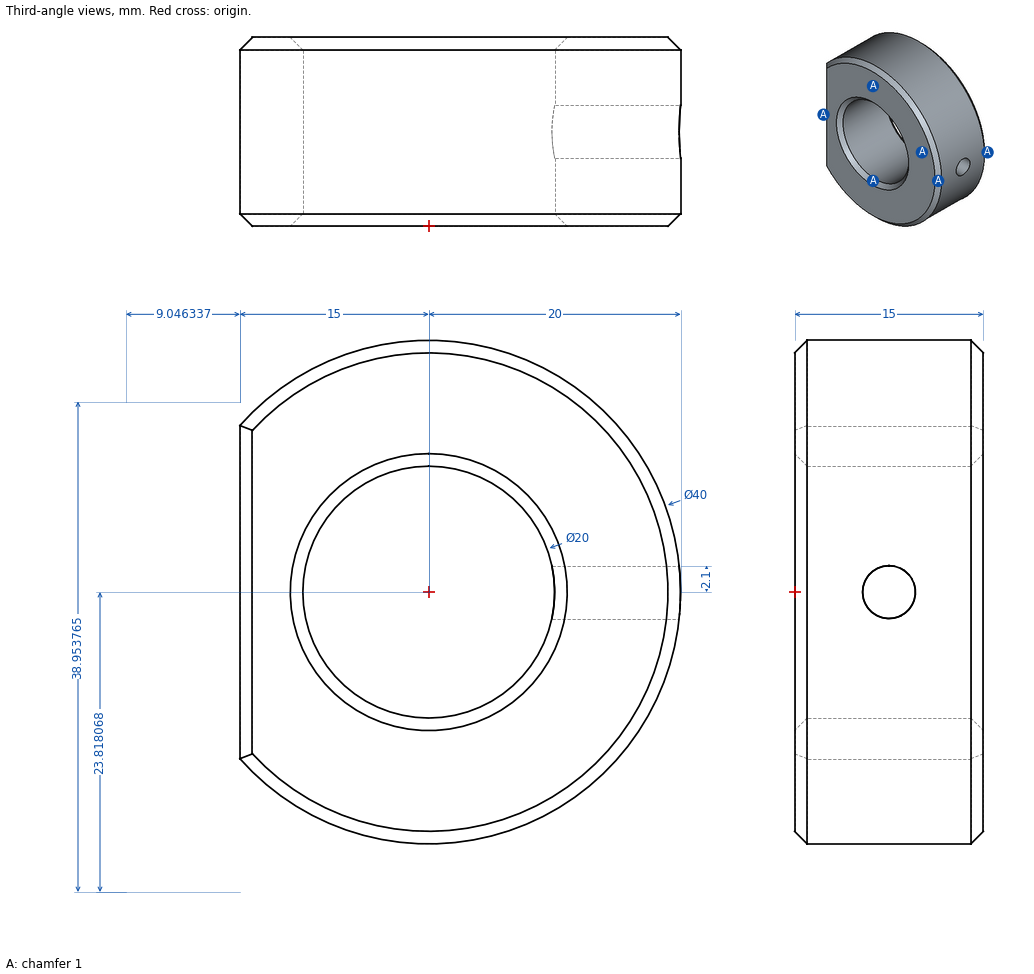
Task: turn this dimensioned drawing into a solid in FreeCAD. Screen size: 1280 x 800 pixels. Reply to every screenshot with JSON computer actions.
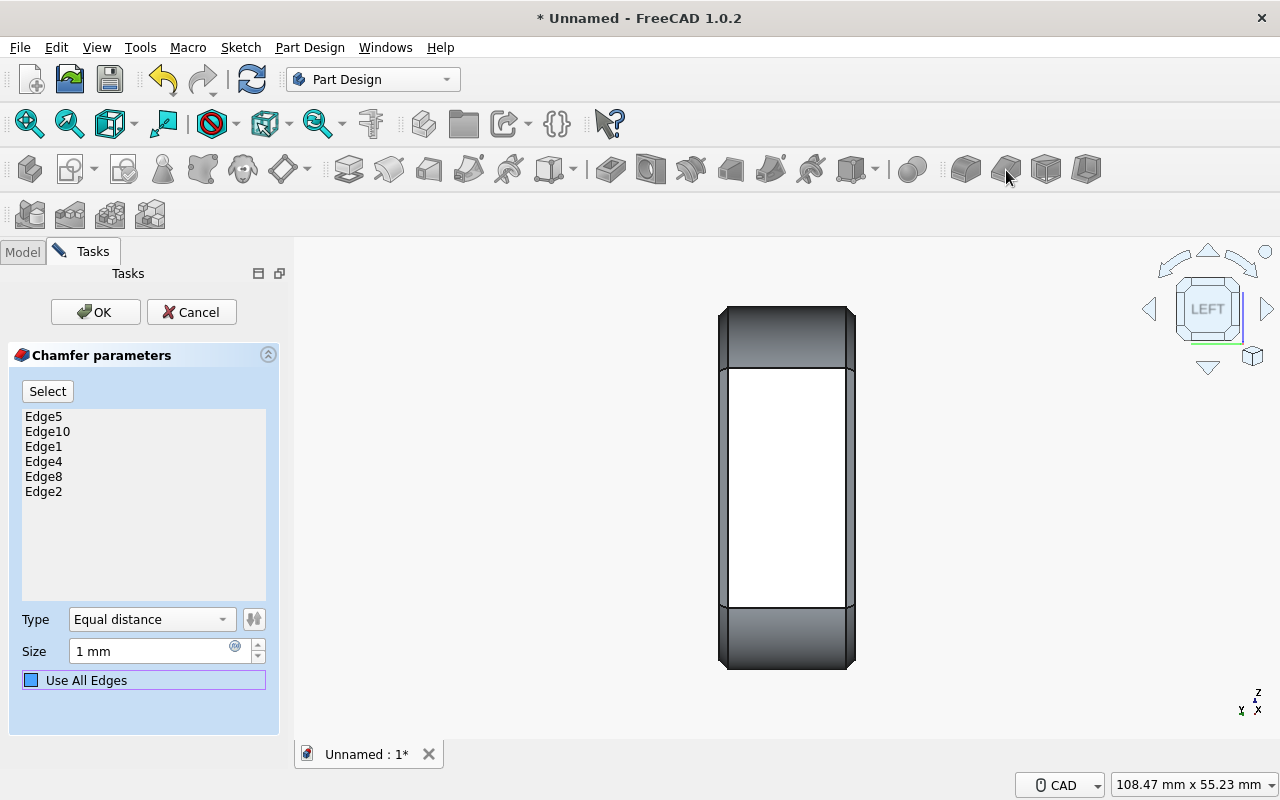
{"action": "left_click", "coordinate": [96, 312]}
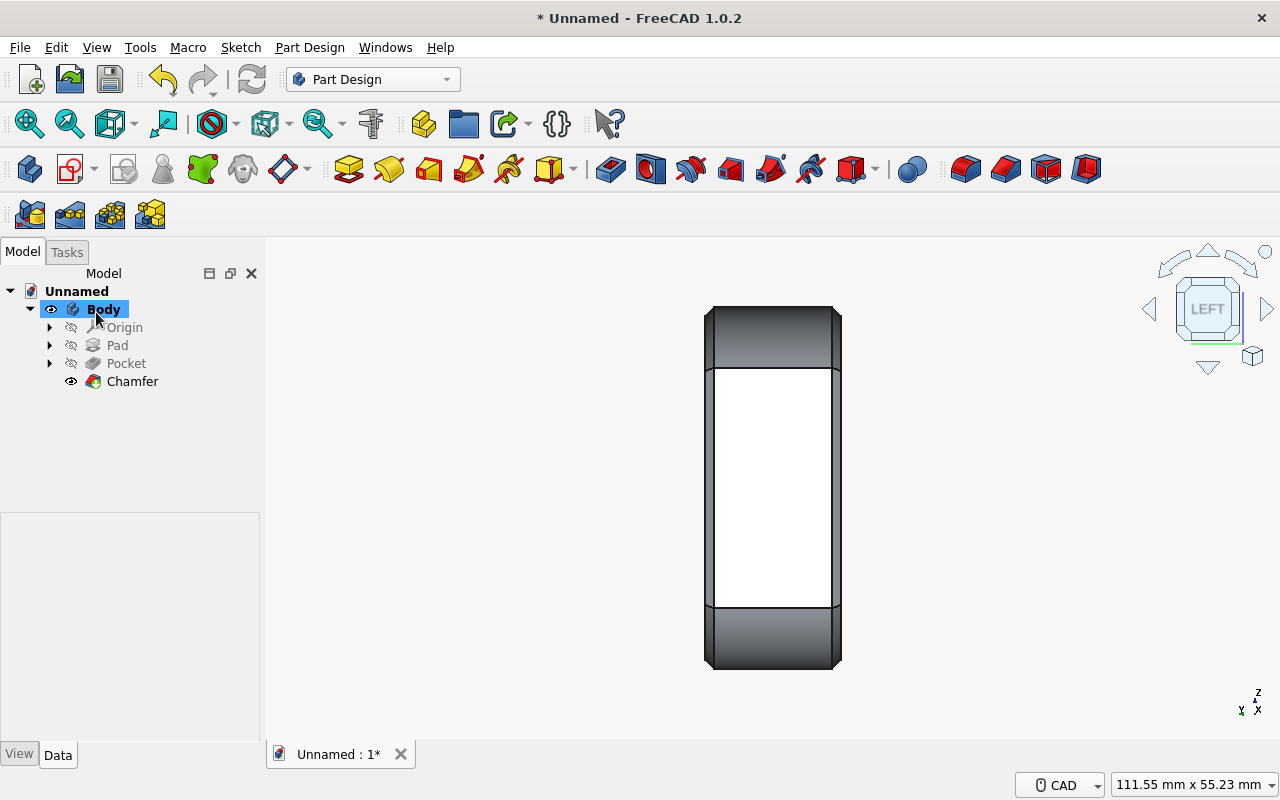
{"action": "left_click", "coordinate": [50, 327]}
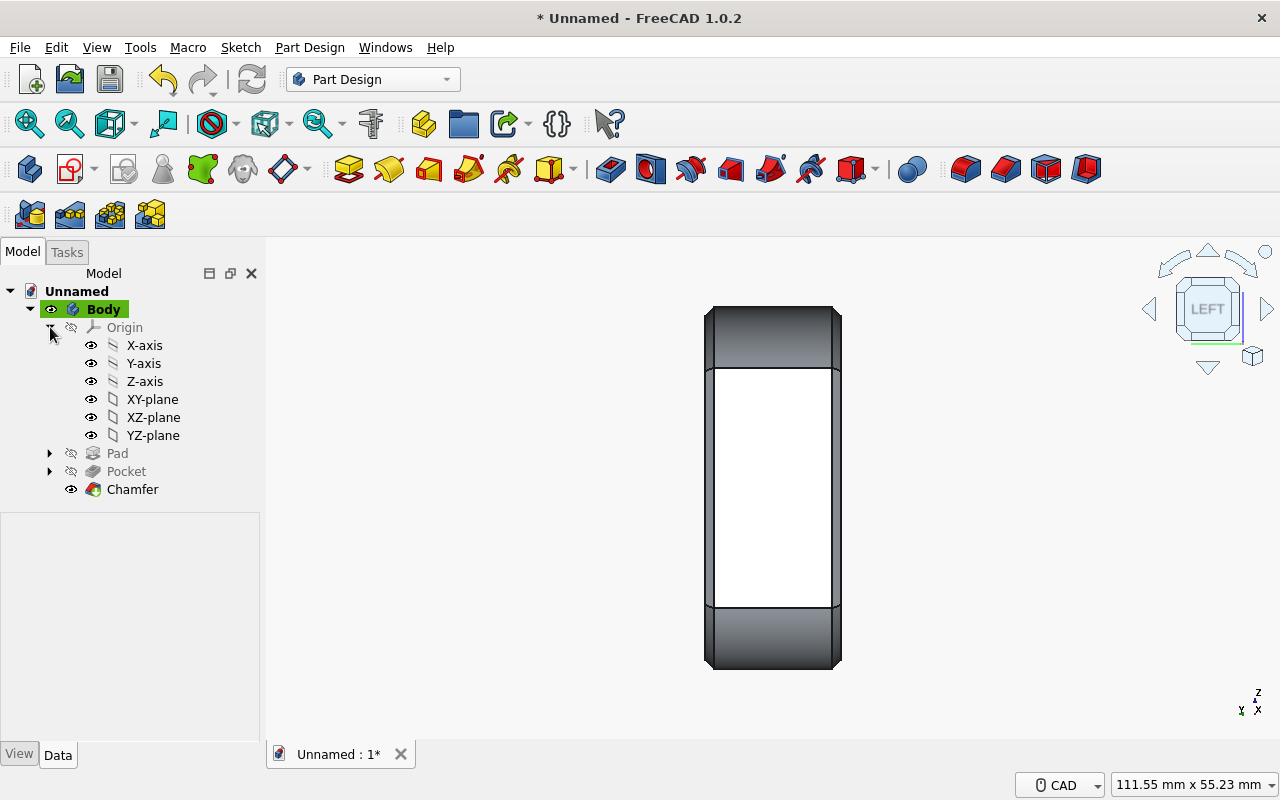
{"action": "left_click", "coordinate": [136, 417]}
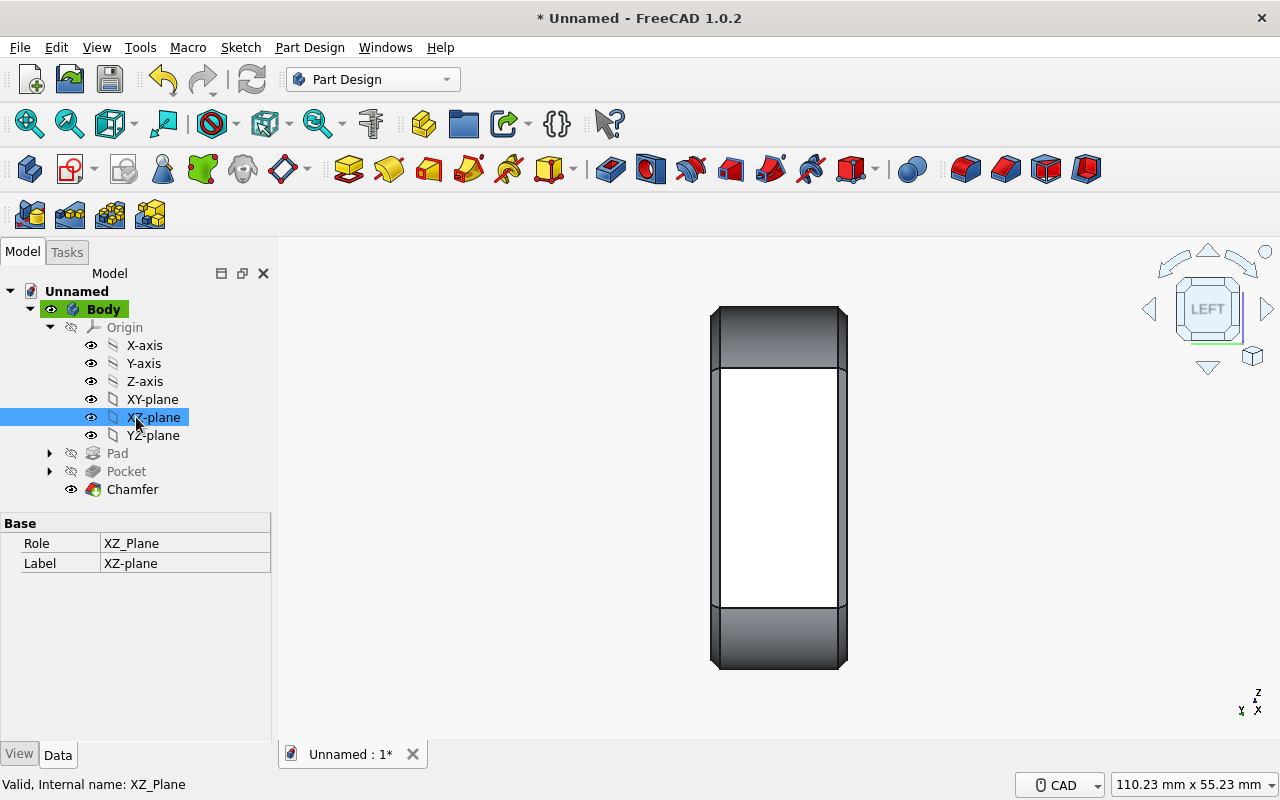
{"action": "left_click", "coordinate": [284, 170]}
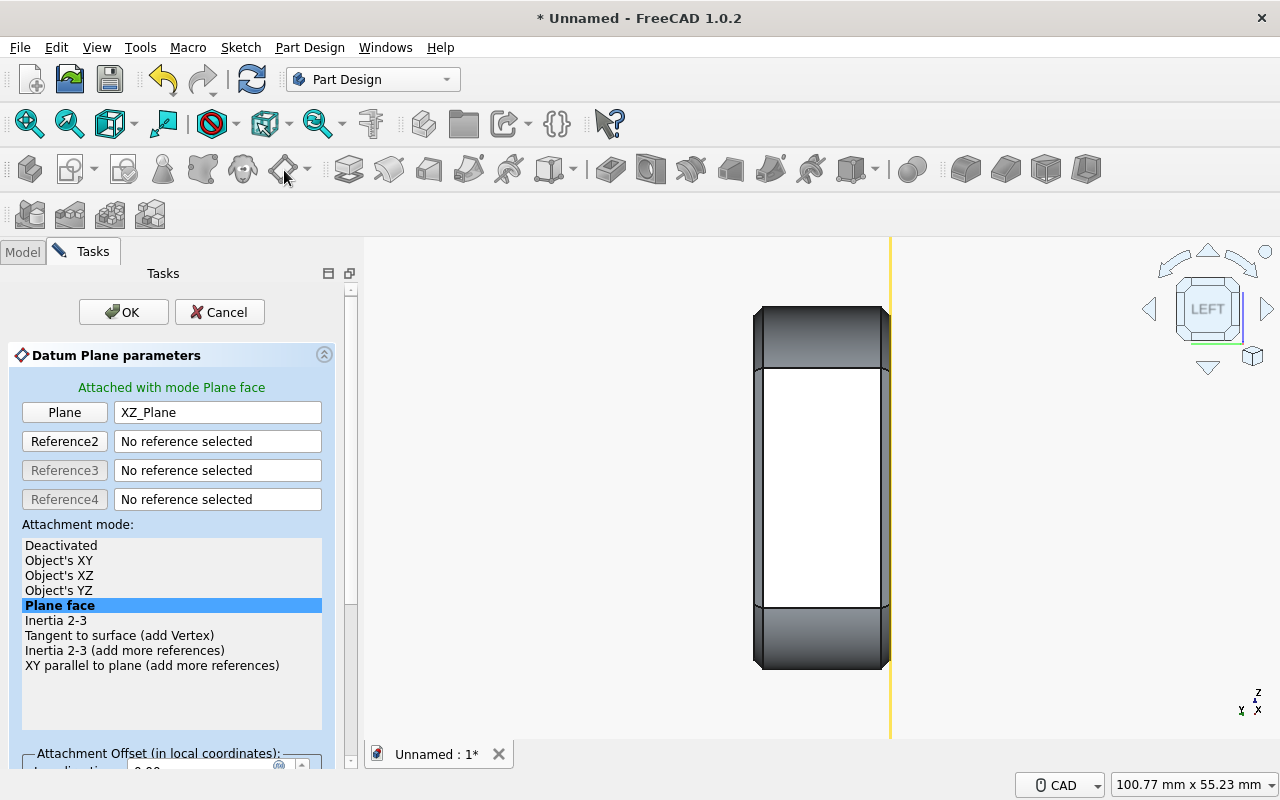
{"action": "scroll", "coordinate": [351, 526], "scroll_direction": "down", "scroll_amount": 3}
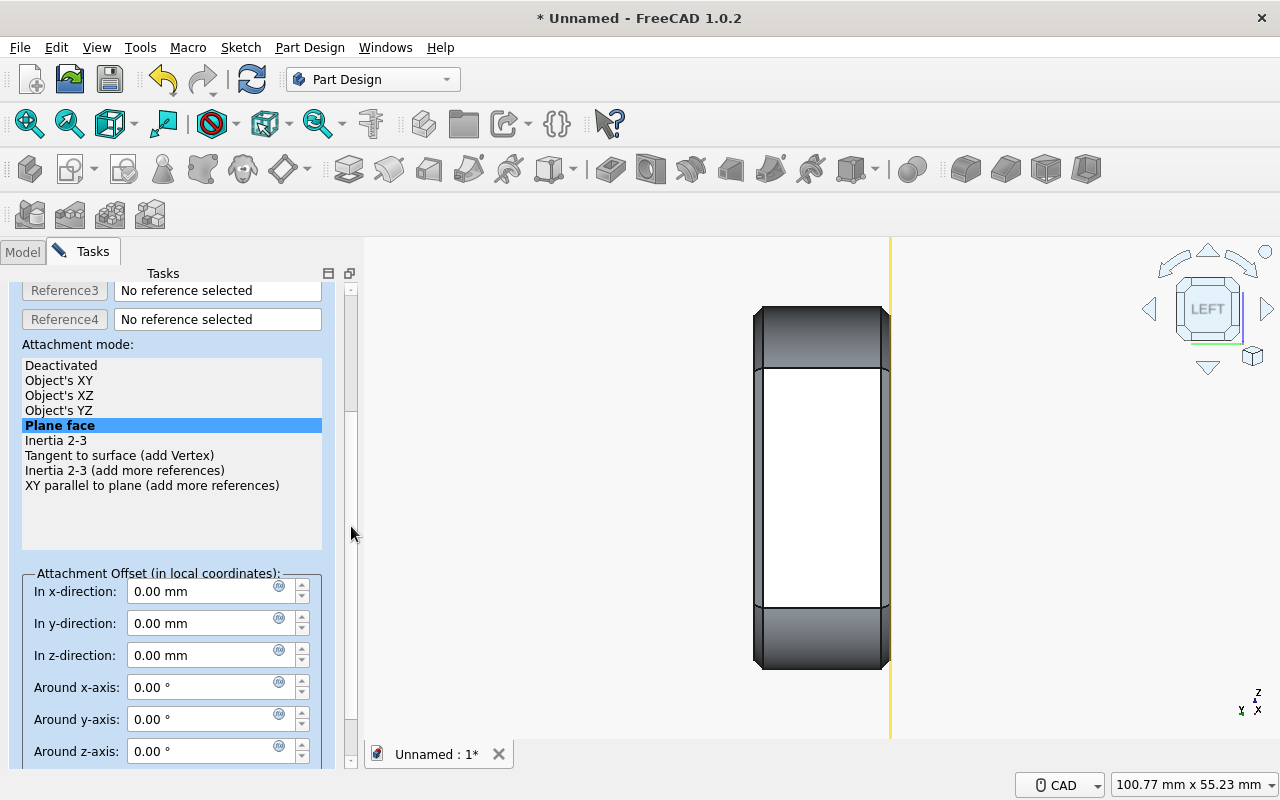
{"action": "triple_click", "coordinate": [210, 655]}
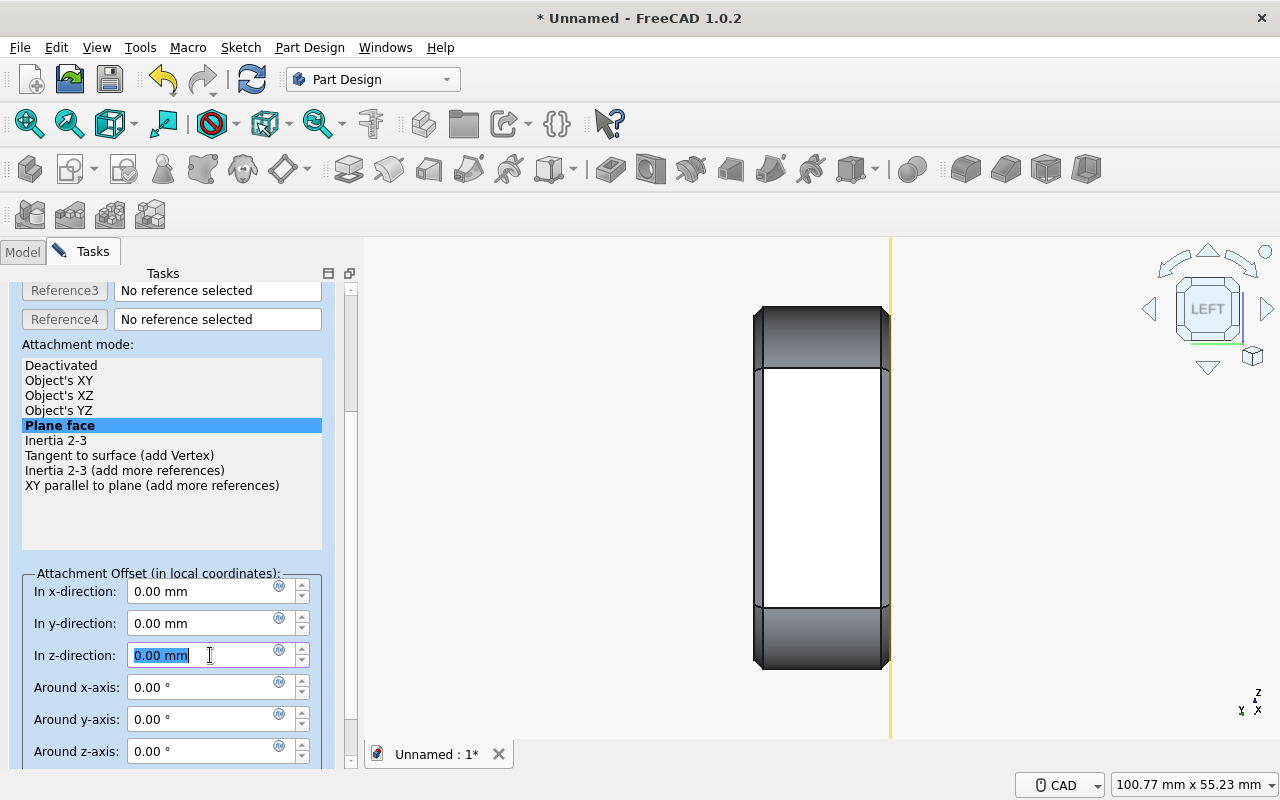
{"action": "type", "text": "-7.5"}
{"action": "key", "text": "Tab"}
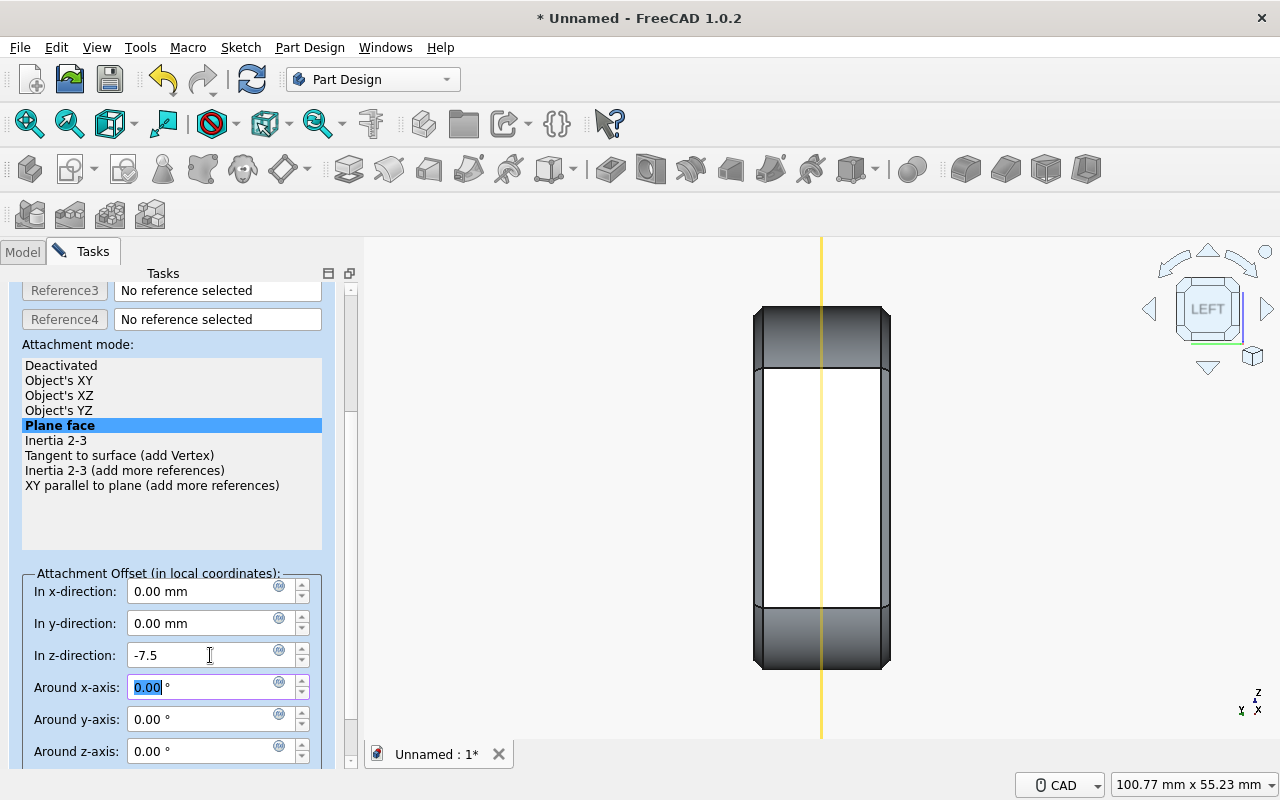
{"action": "scroll", "coordinate": [351, 526], "scroll_direction": "up", "scroll_amount": 4}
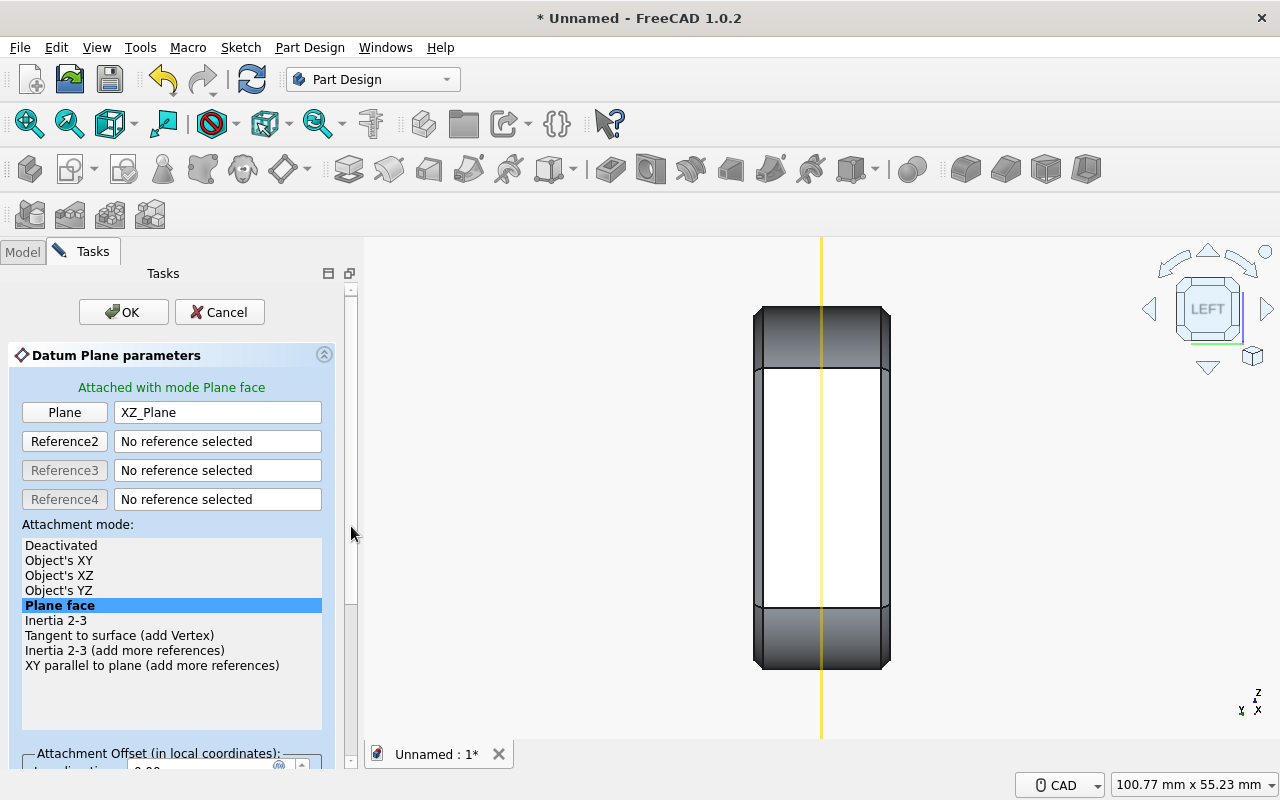
{"action": "left_click", "coordinate": [124, 312]}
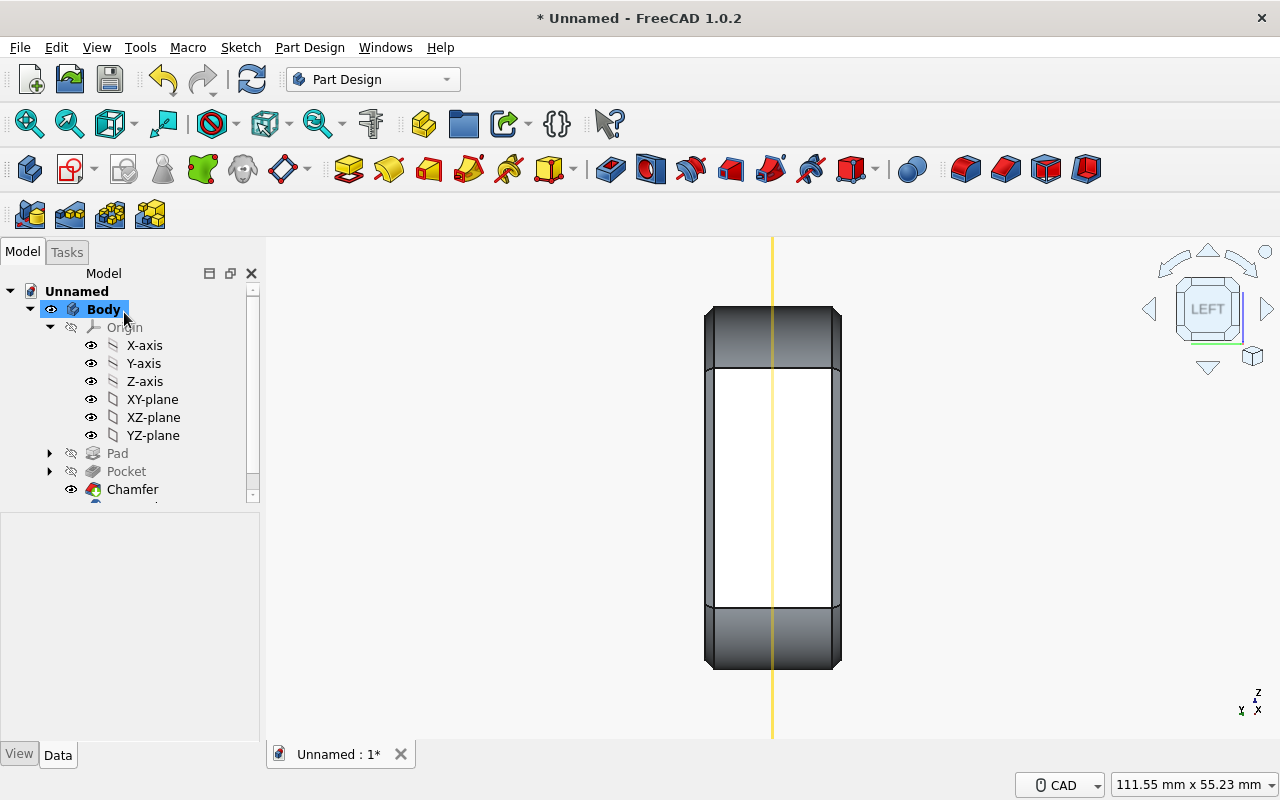
{"action": "scroll", "coordinate": [100, 395], "scroll_direction": "down", "scroll_amount": 3}